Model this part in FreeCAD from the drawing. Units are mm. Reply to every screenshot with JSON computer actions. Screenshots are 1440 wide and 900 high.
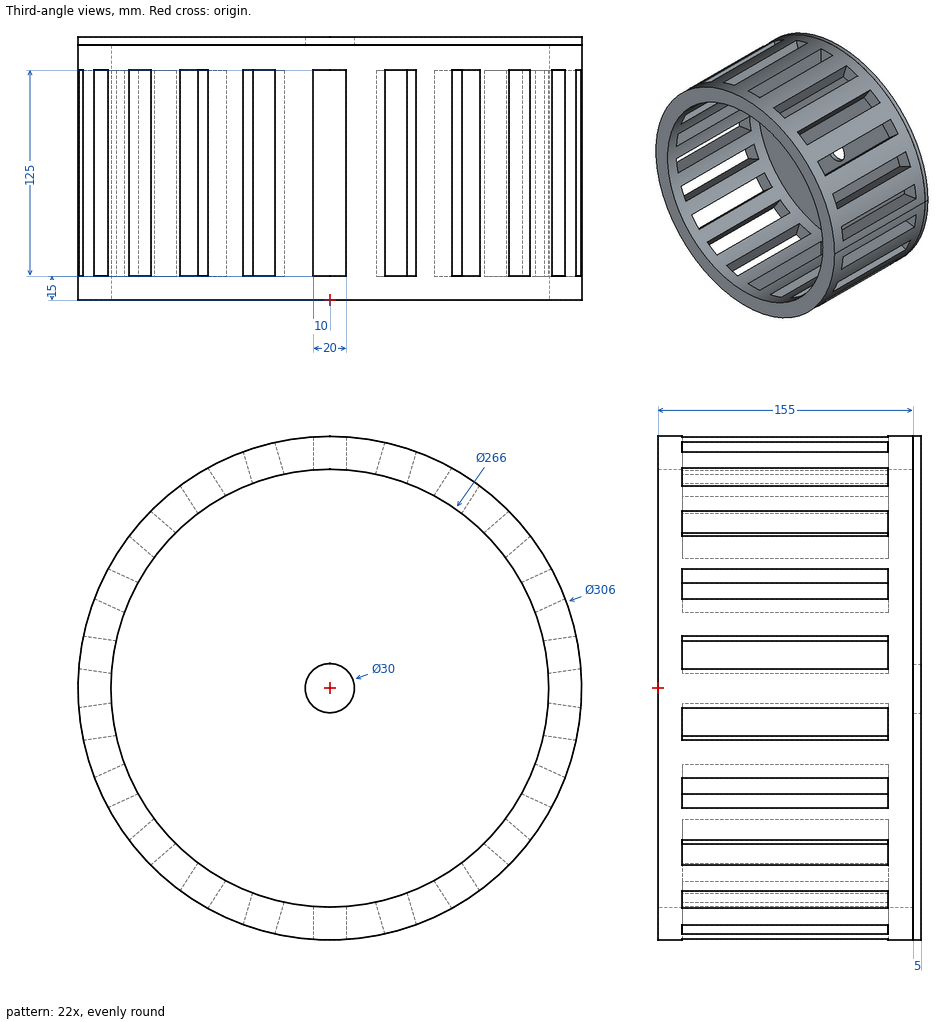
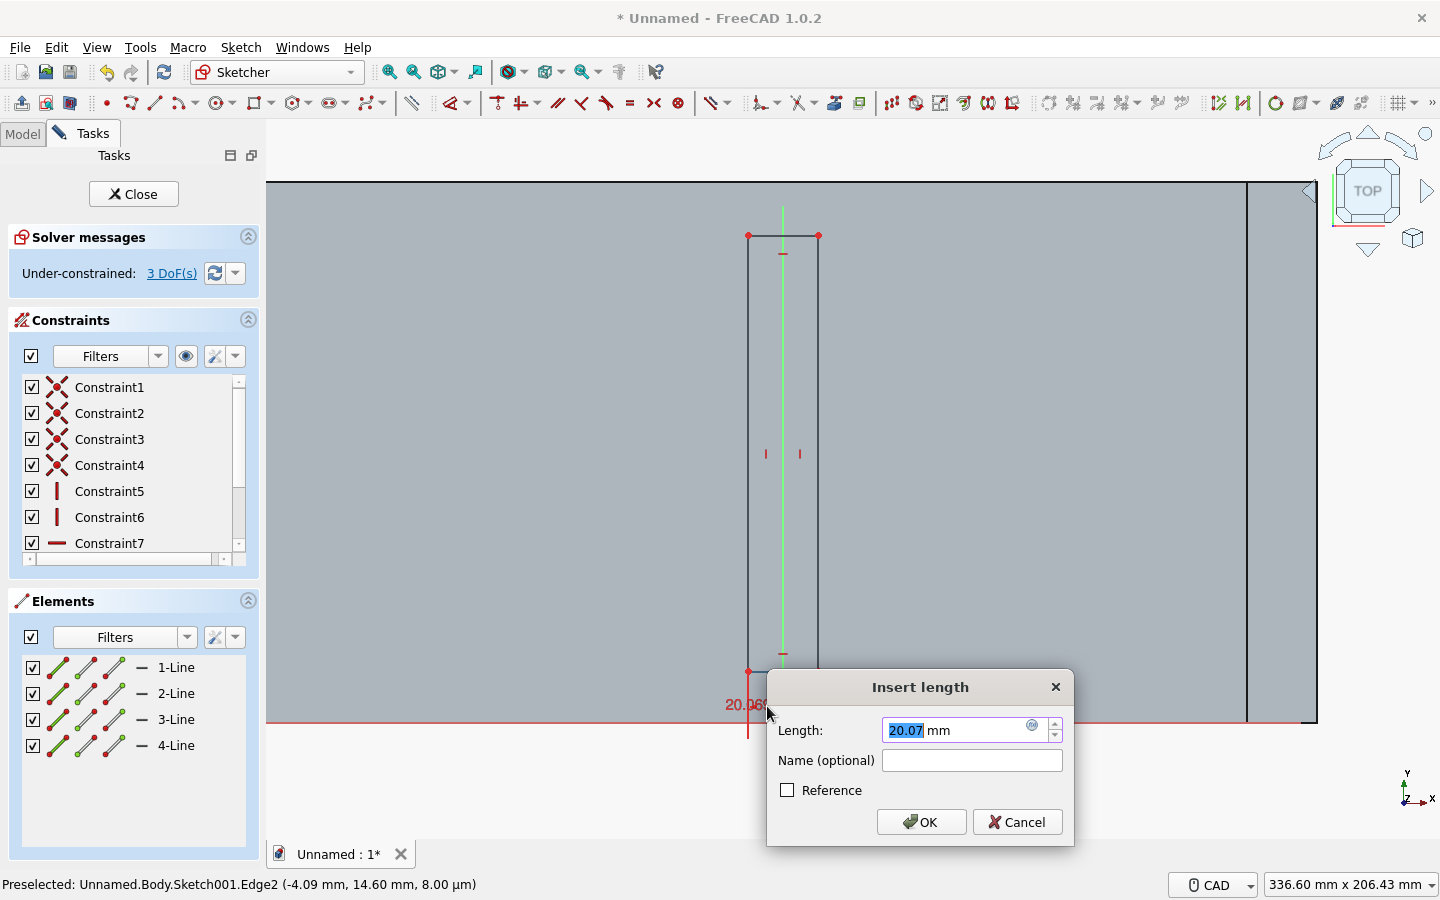
{"action": "type", "text": "20"}
{"action": "key", "text": "Return"}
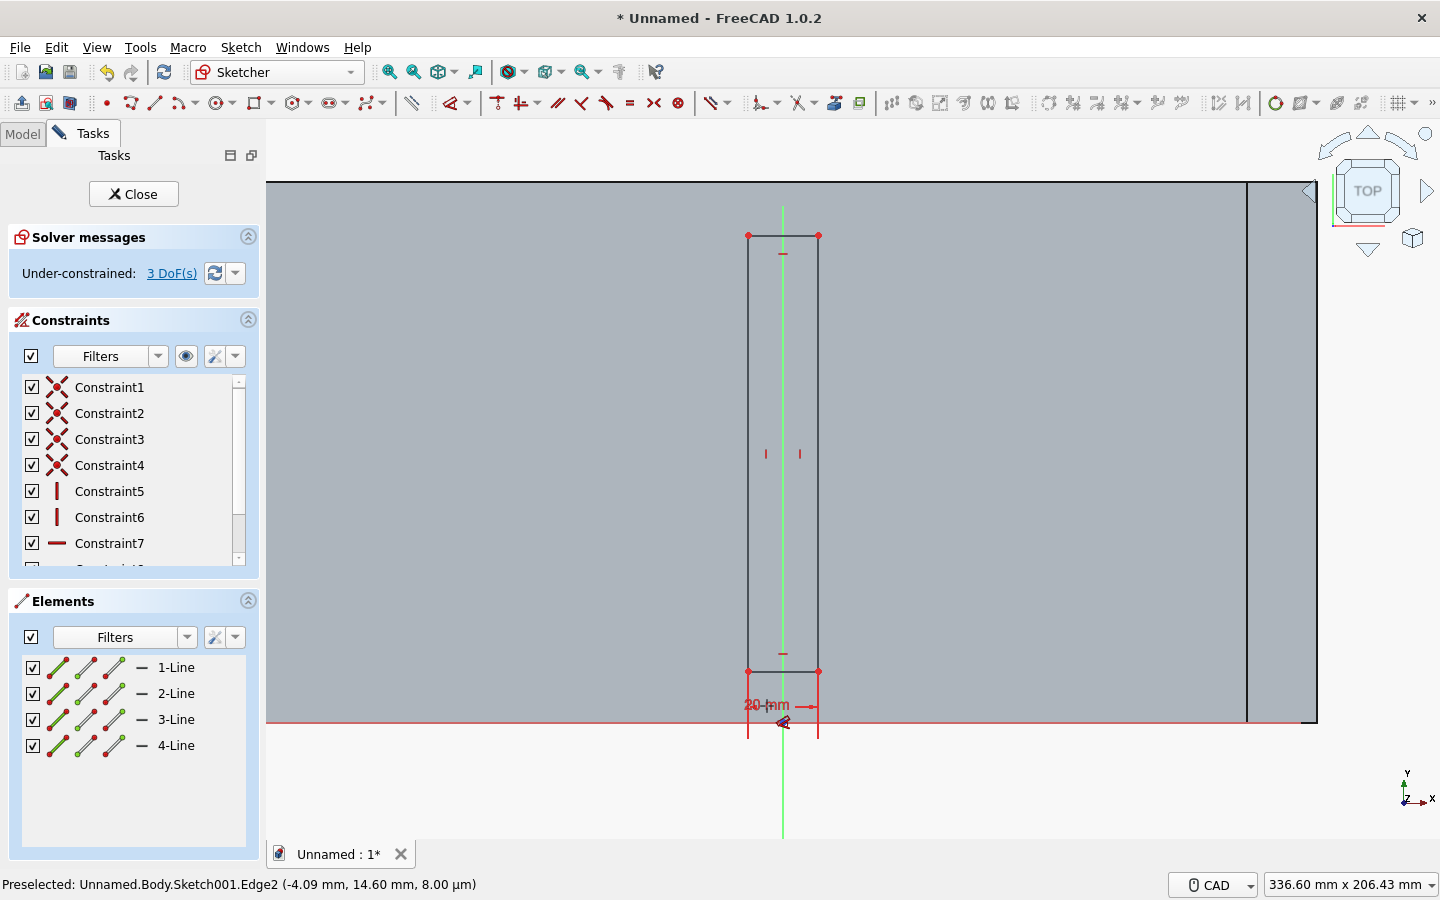
{"action": "left_click", "coordinate": [748, 367]}
{"action": "left_click", "coordinate": [714, 454]}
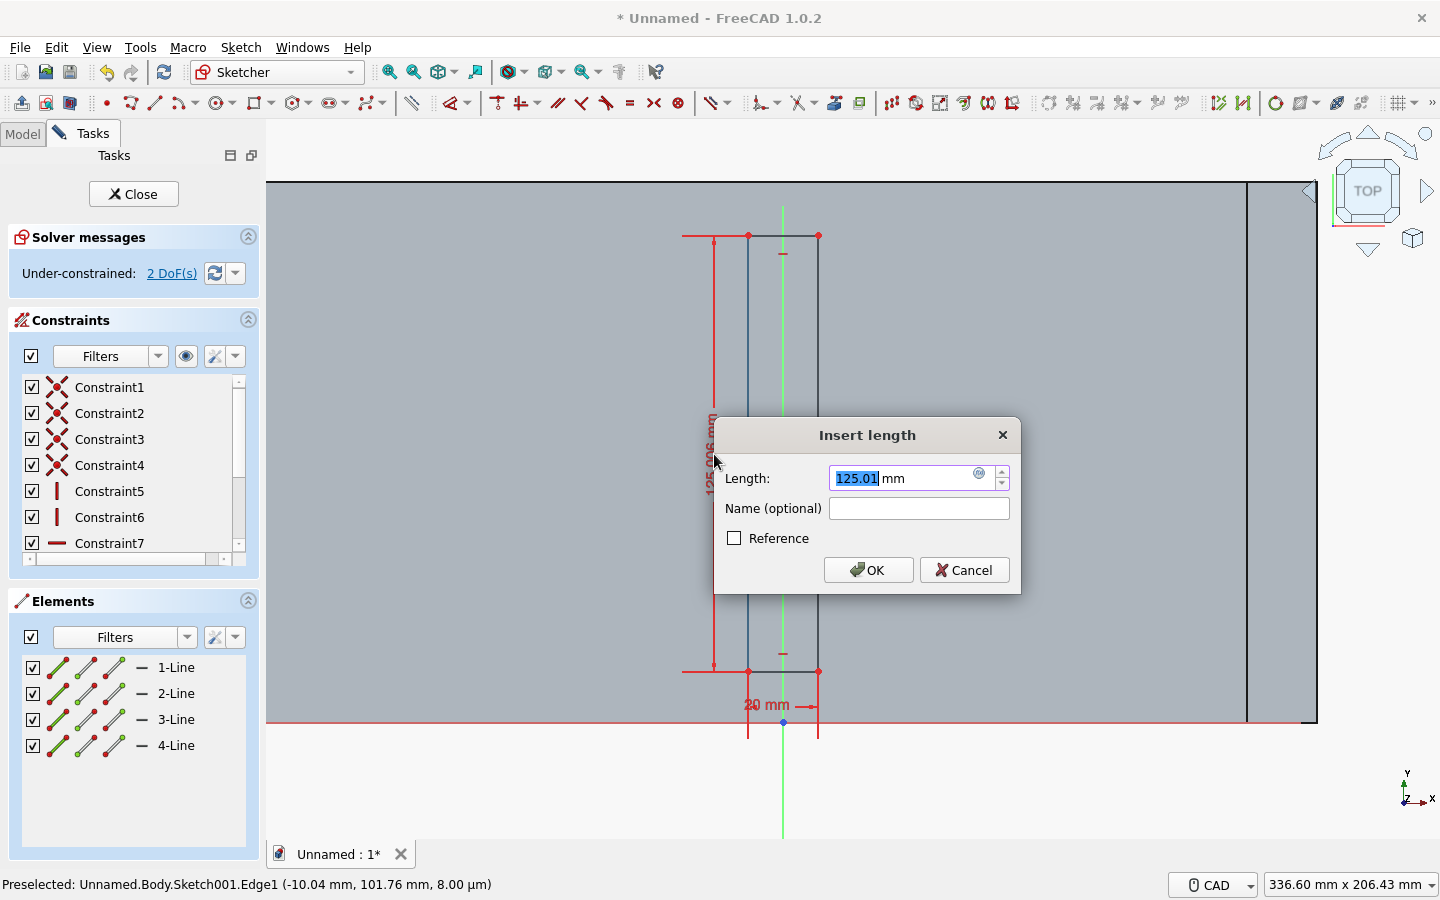
{"action": "type", "text": "125"}
{"action": "key", "text": "Return"}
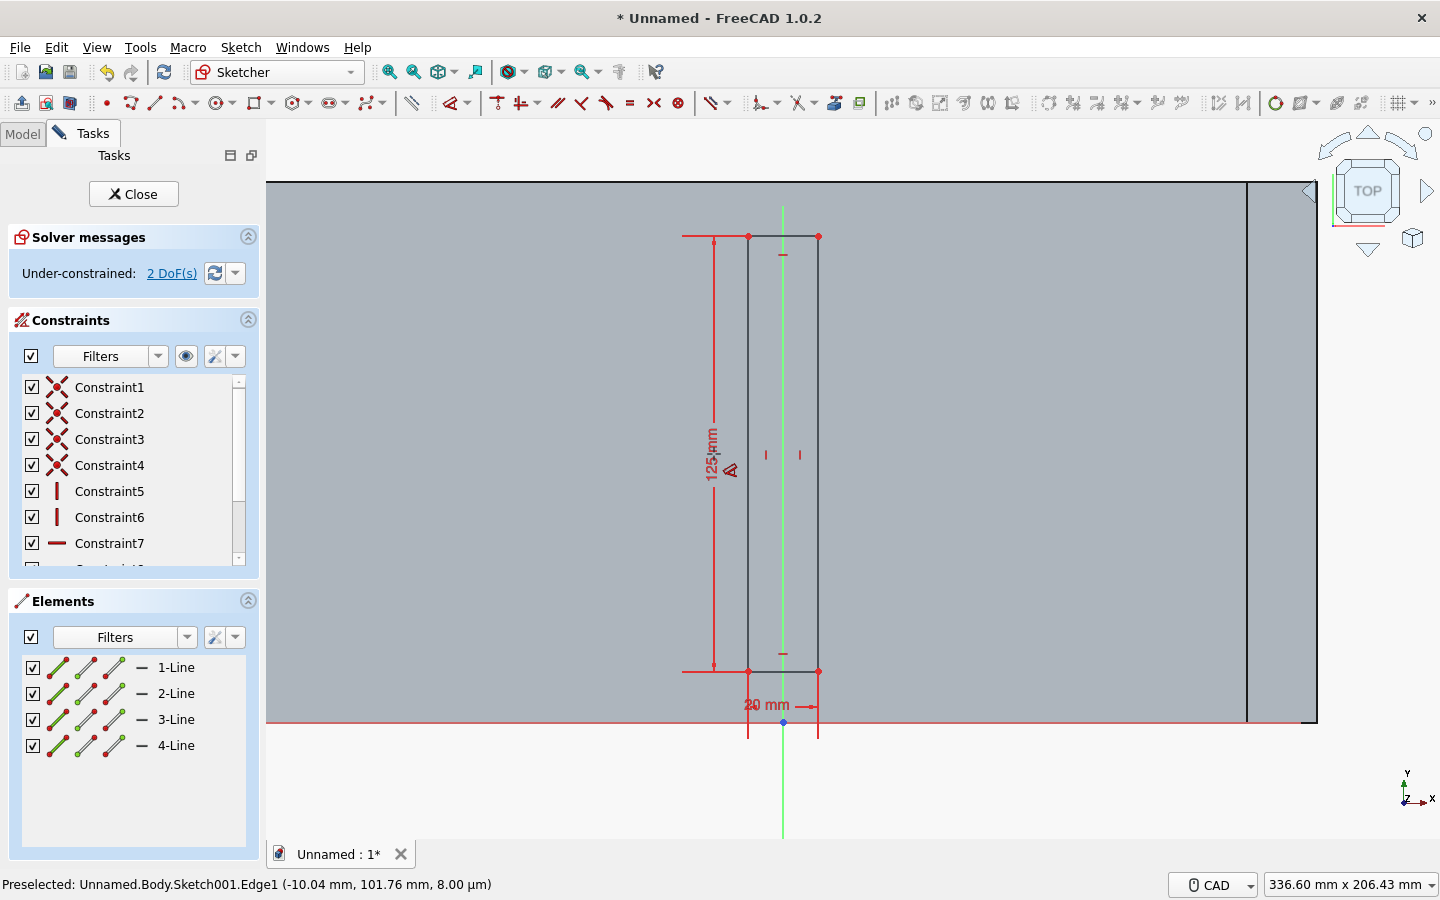
{"action": "left_click", "coordinate": [748, 236]}
{"action": "left_click", "coordinate": [766, 757]}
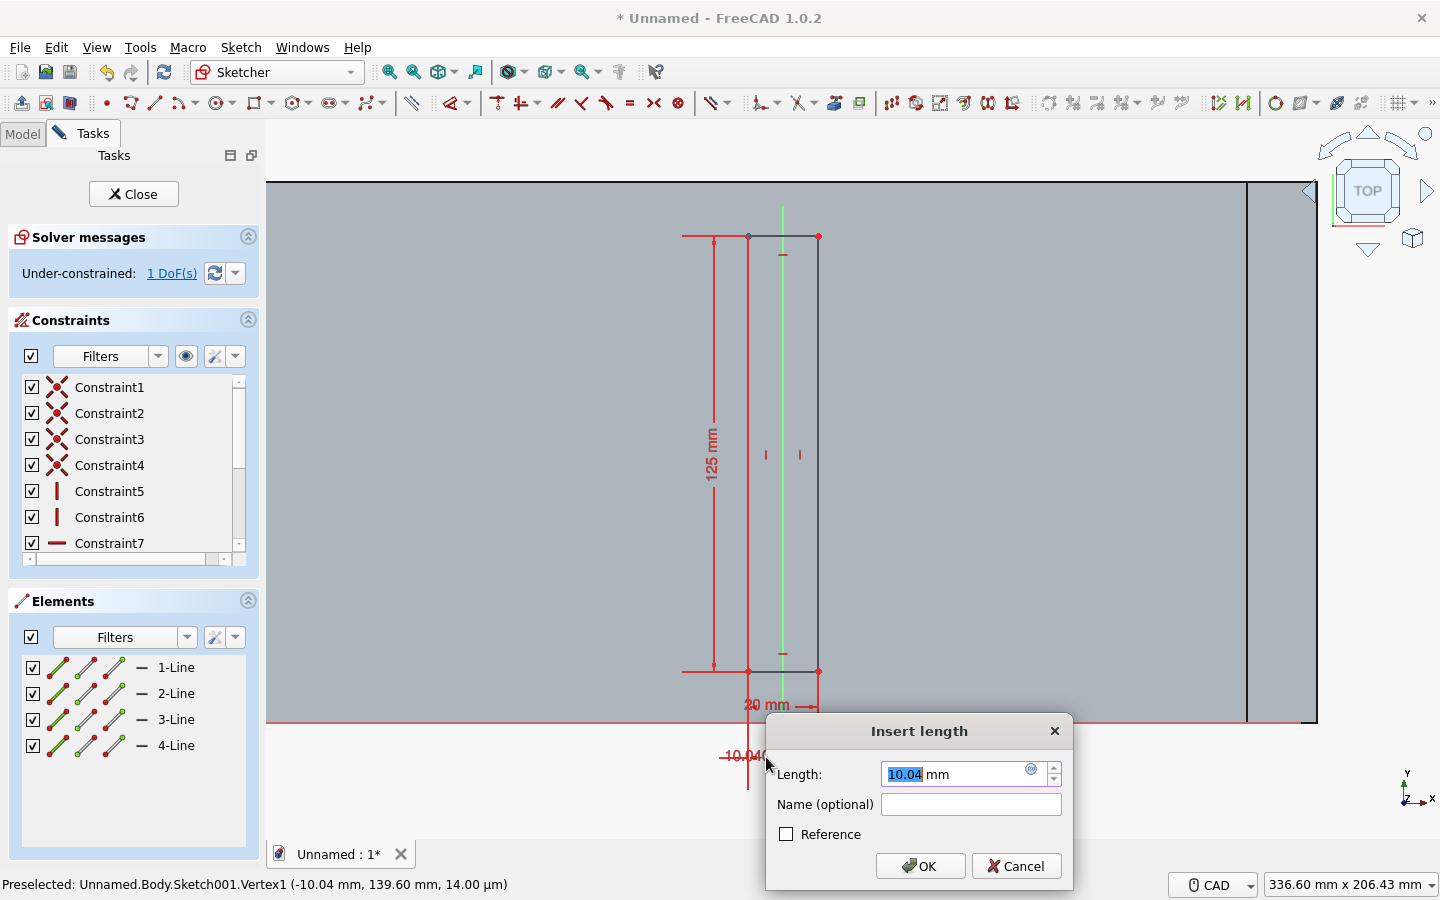
{"action": "type", "text": "10"}
{"action": "key", "text": "Return"}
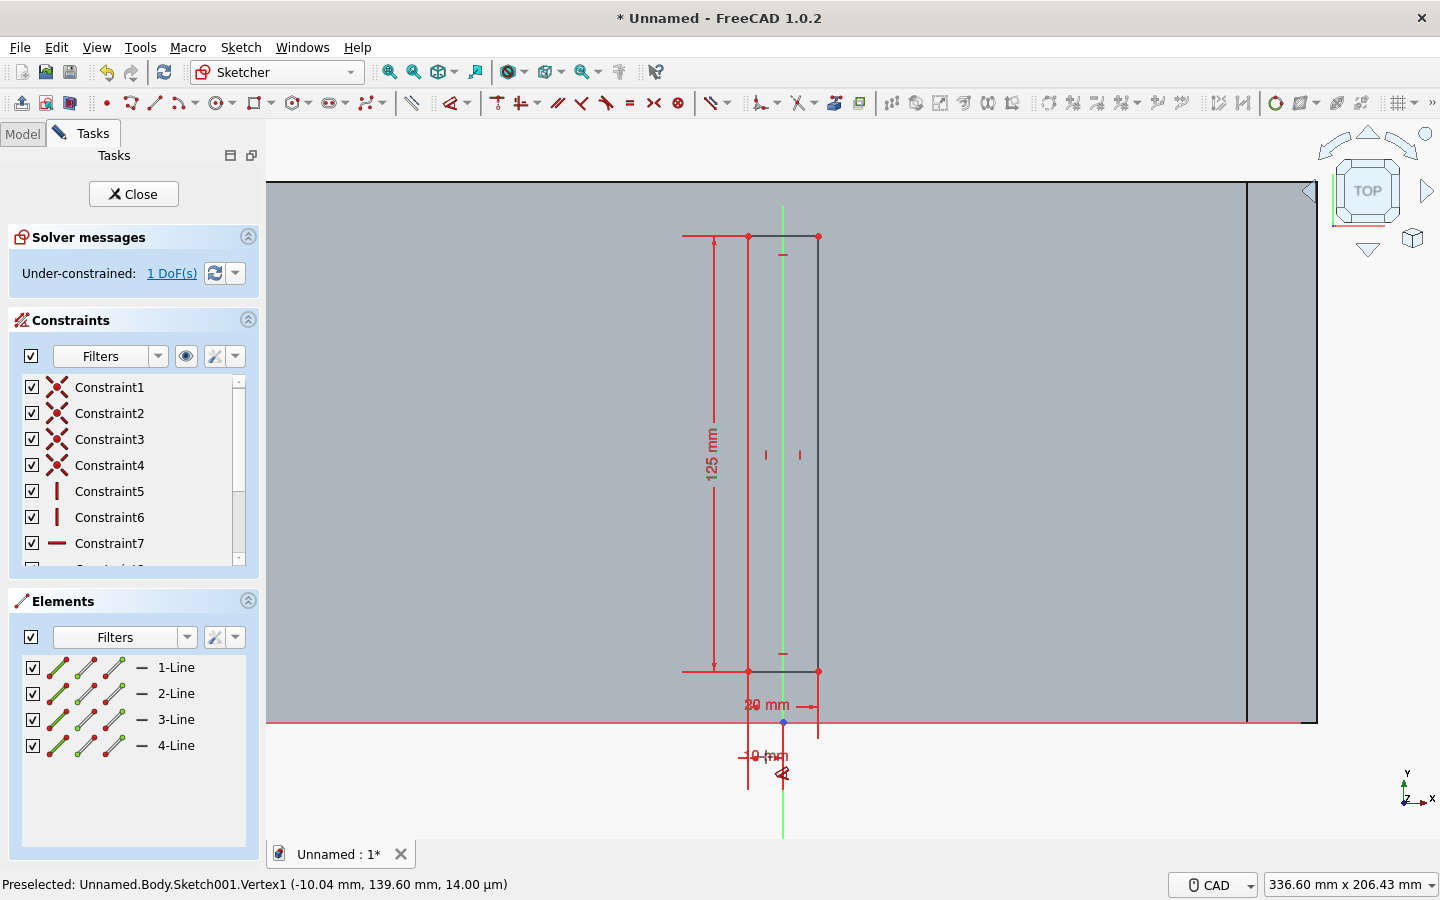
{"action": "left_click", "coordinate": [748, 672]}
{"action": "left_click", "coordinate": [714, 686]}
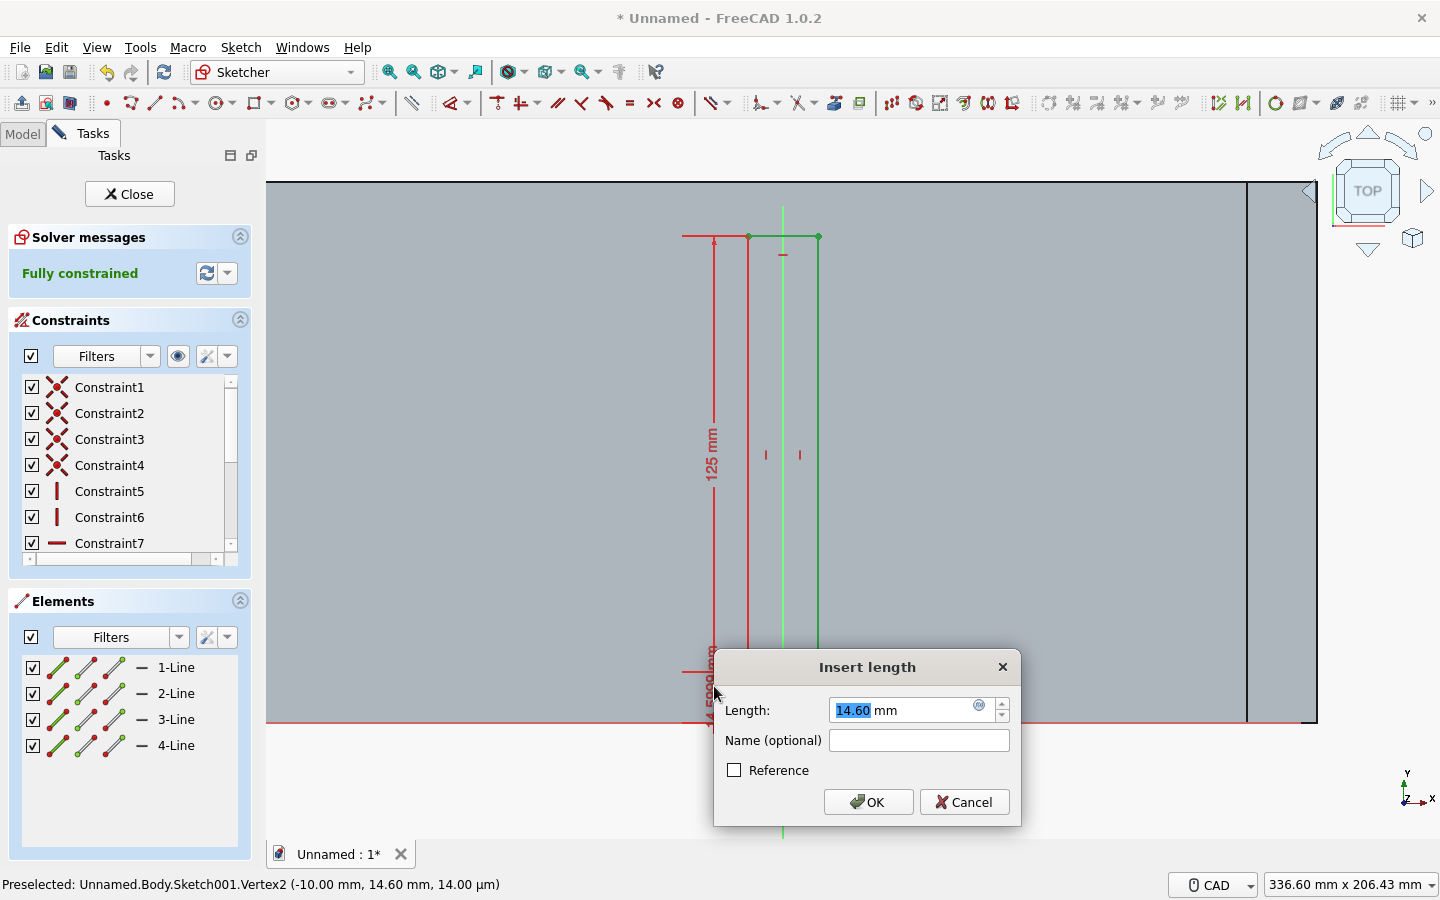
{"action": "type", "text": "15"}
{"action": "key", "text": "Return"}
{"action": "key", "text": "Escape"}